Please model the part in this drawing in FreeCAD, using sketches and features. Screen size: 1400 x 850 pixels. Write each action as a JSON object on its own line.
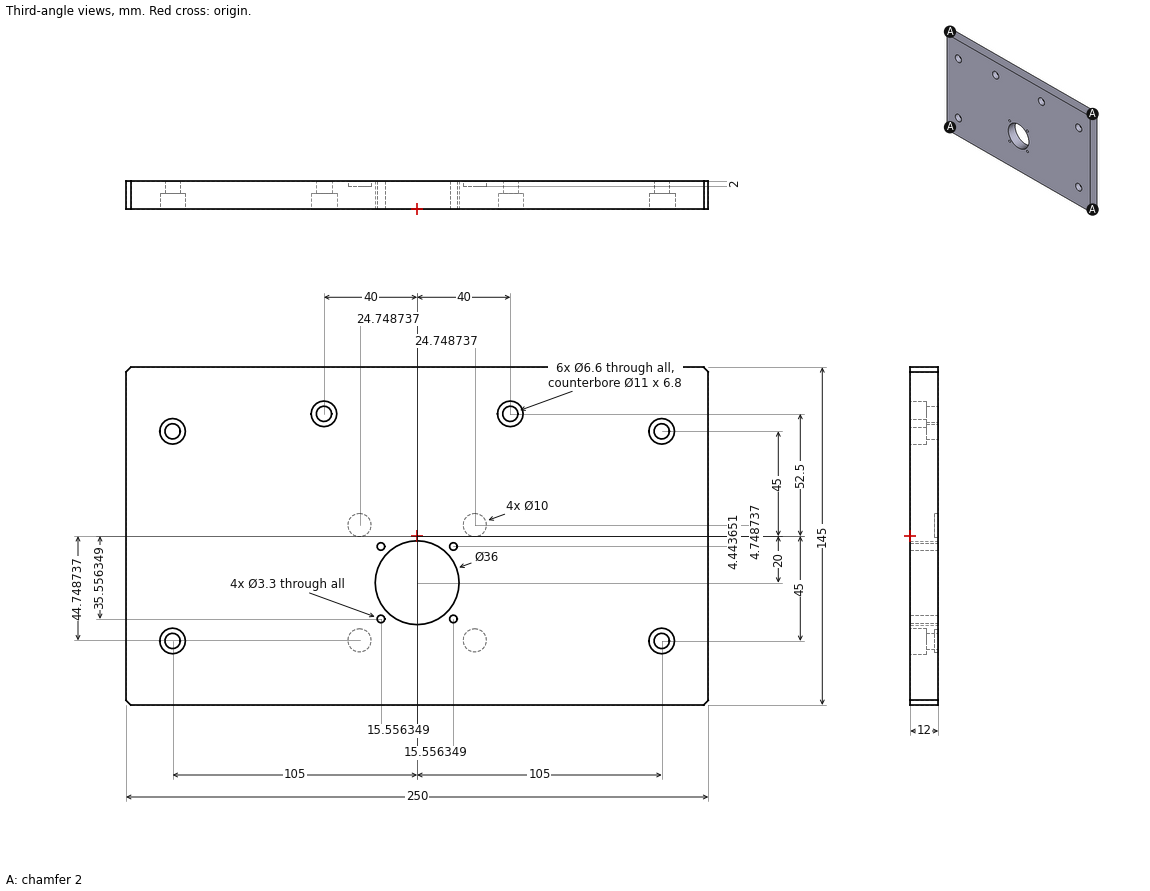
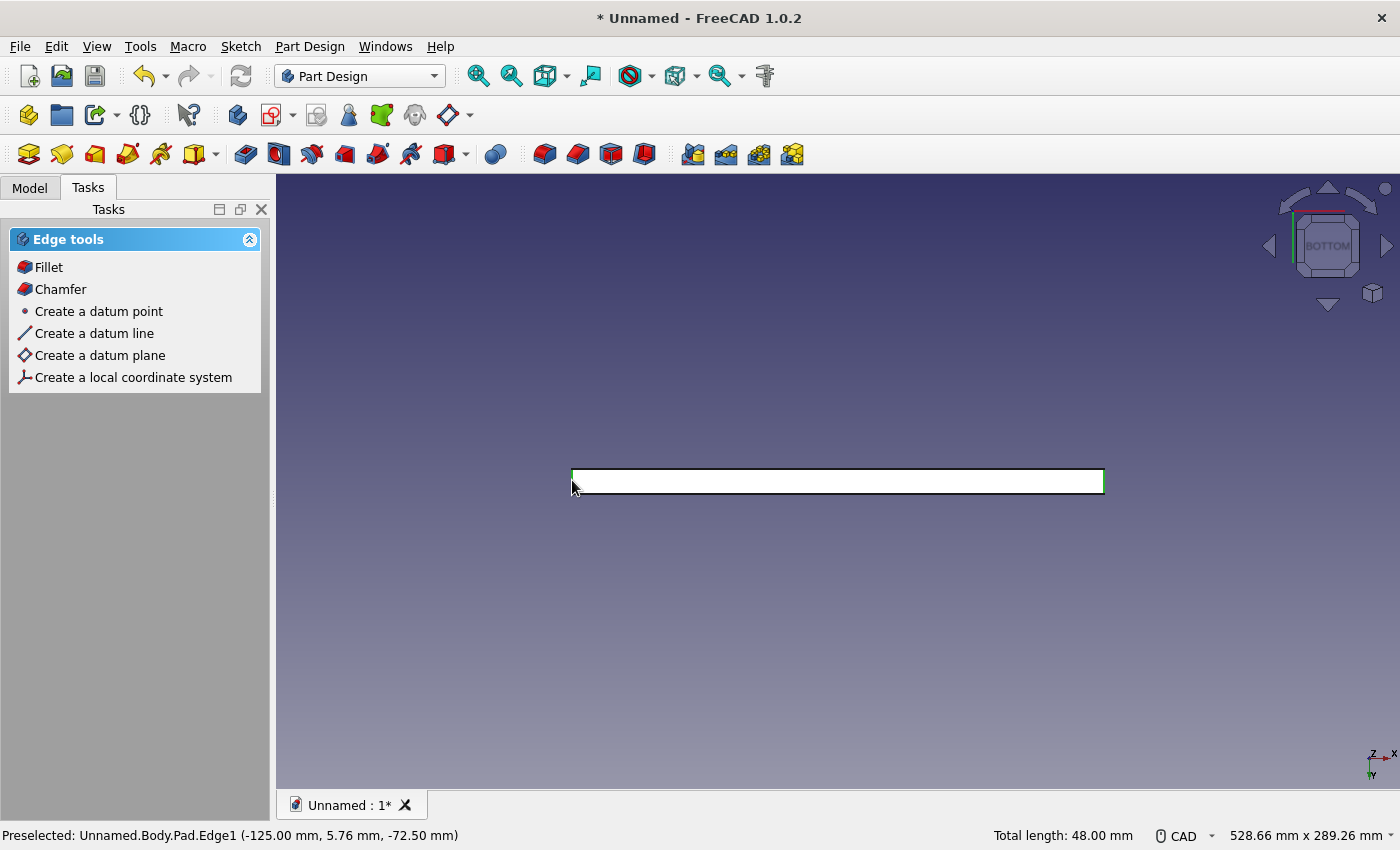
{"action": "left_click", "coordinate": [578, 154]}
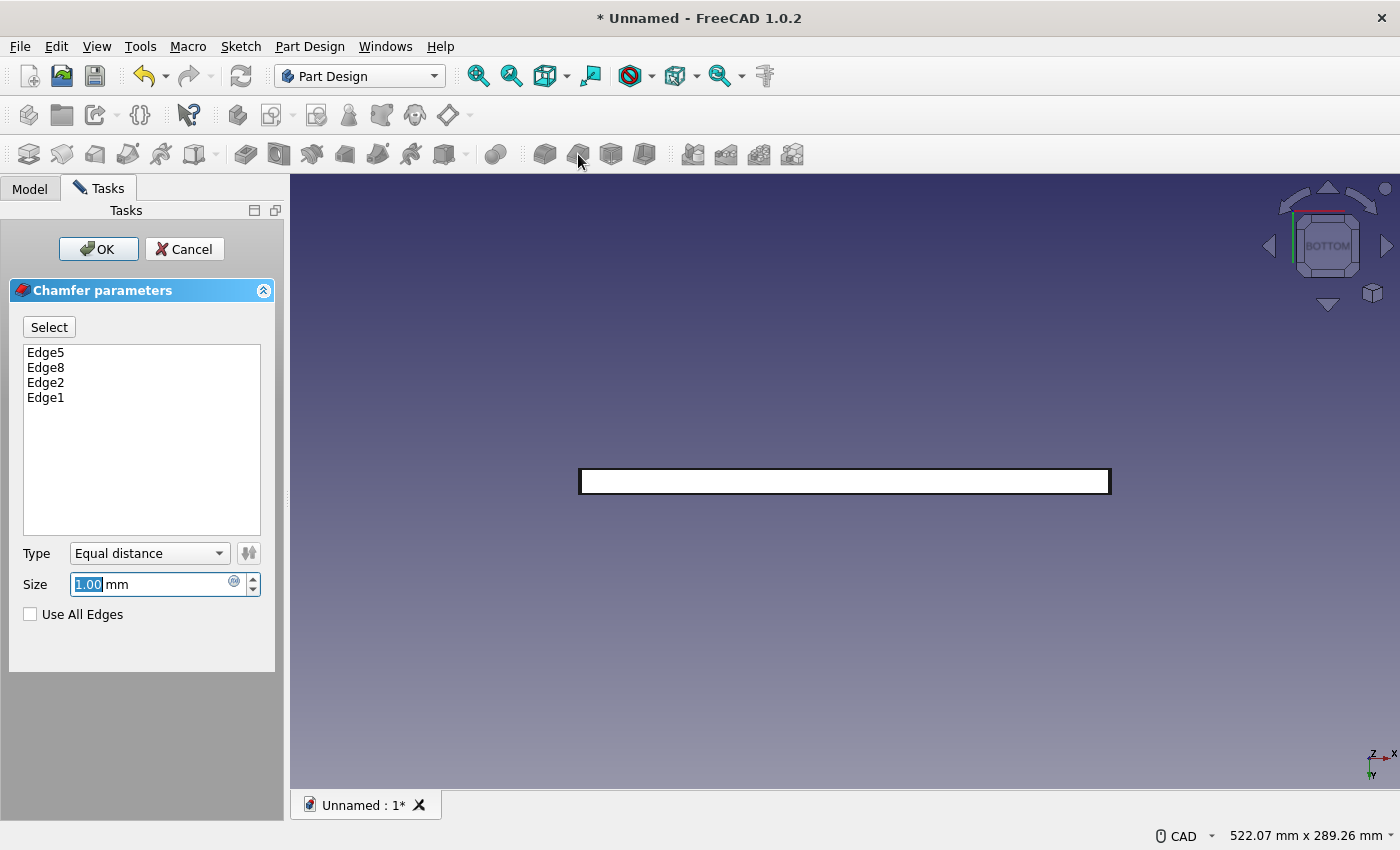
{"action": "type", "text": "2"}
{"action": "key", "text": "Tab"}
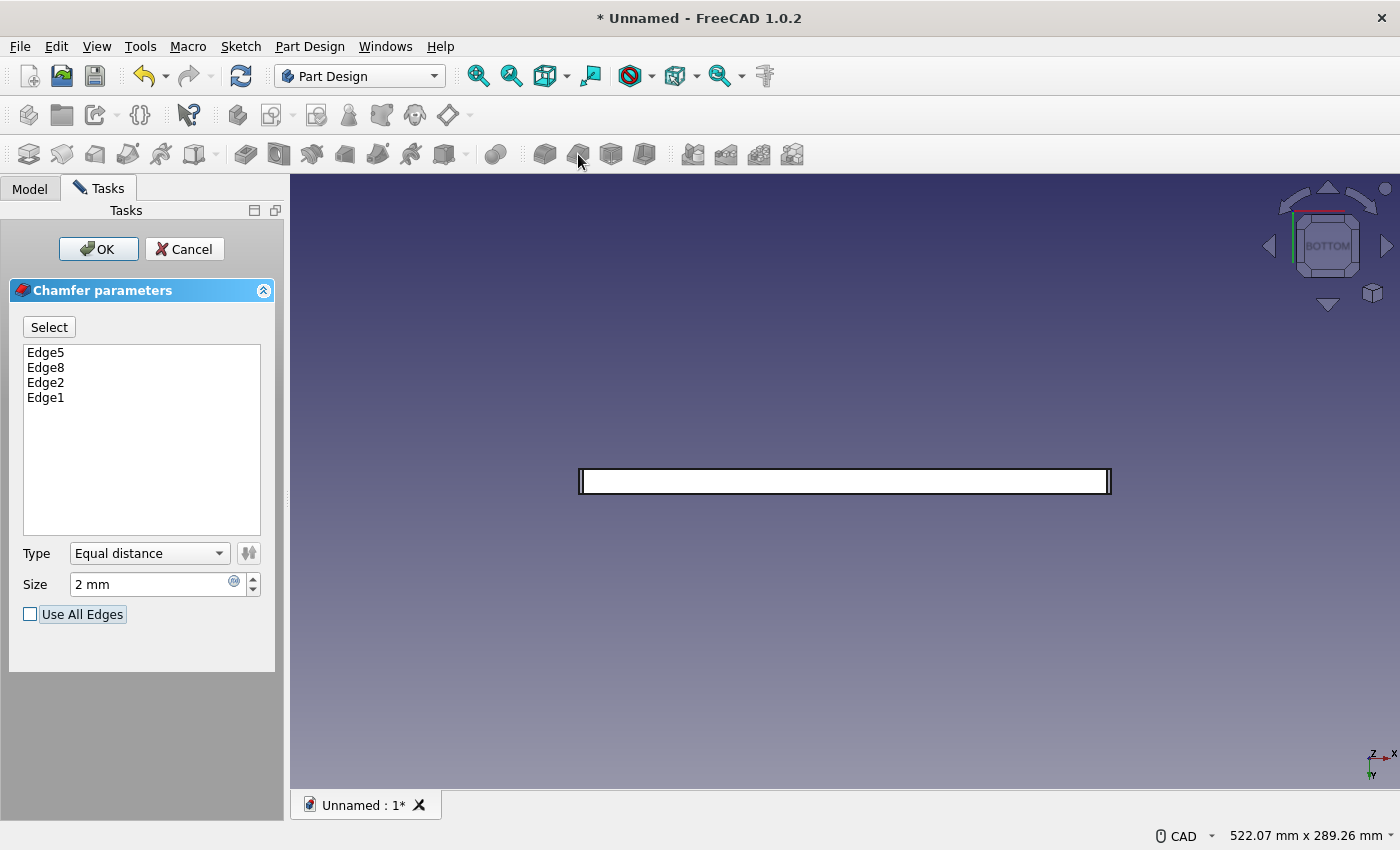
{"action": "left_click", "coordinate": [99, 249]}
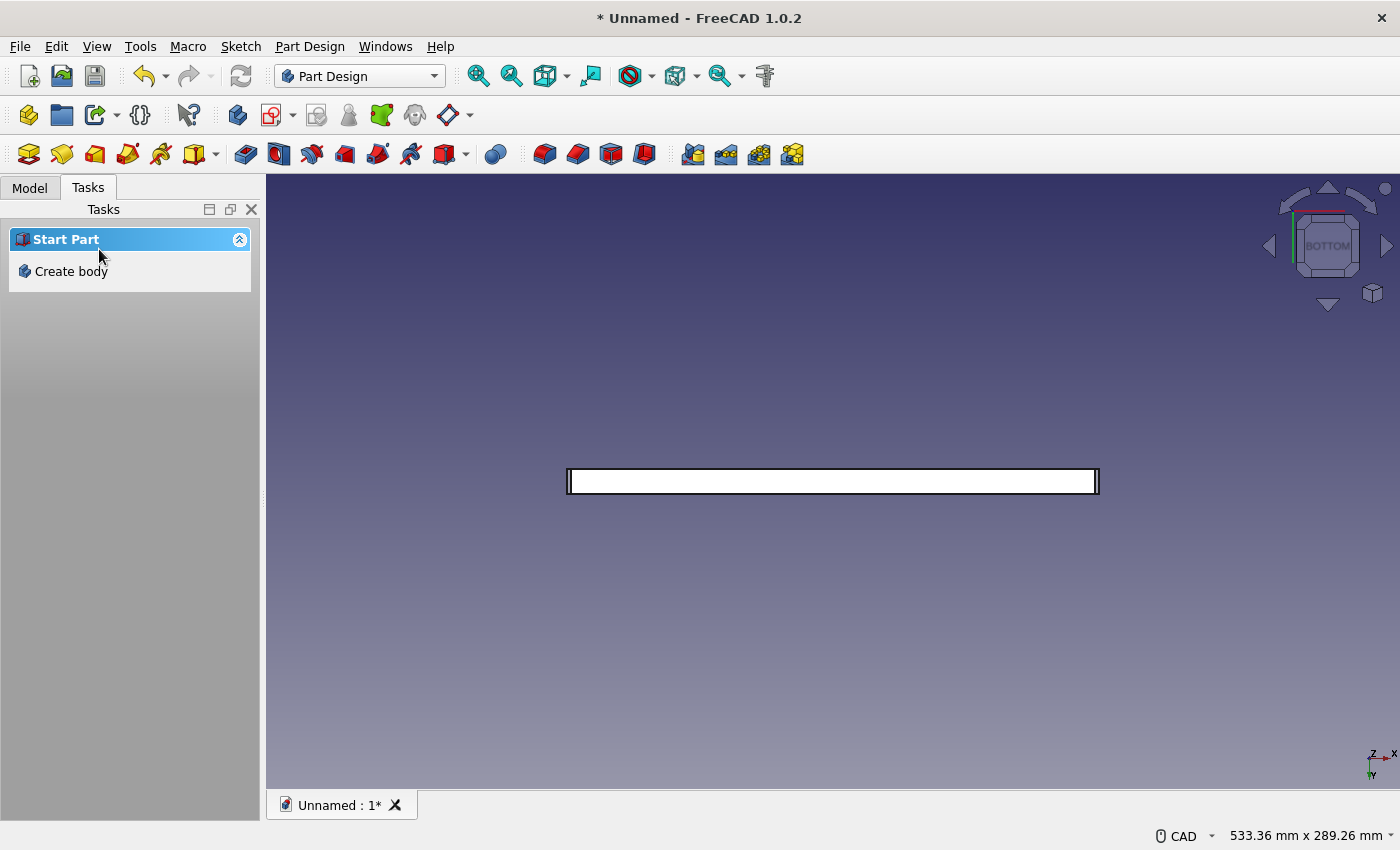
{"action": "key", "text": "4"}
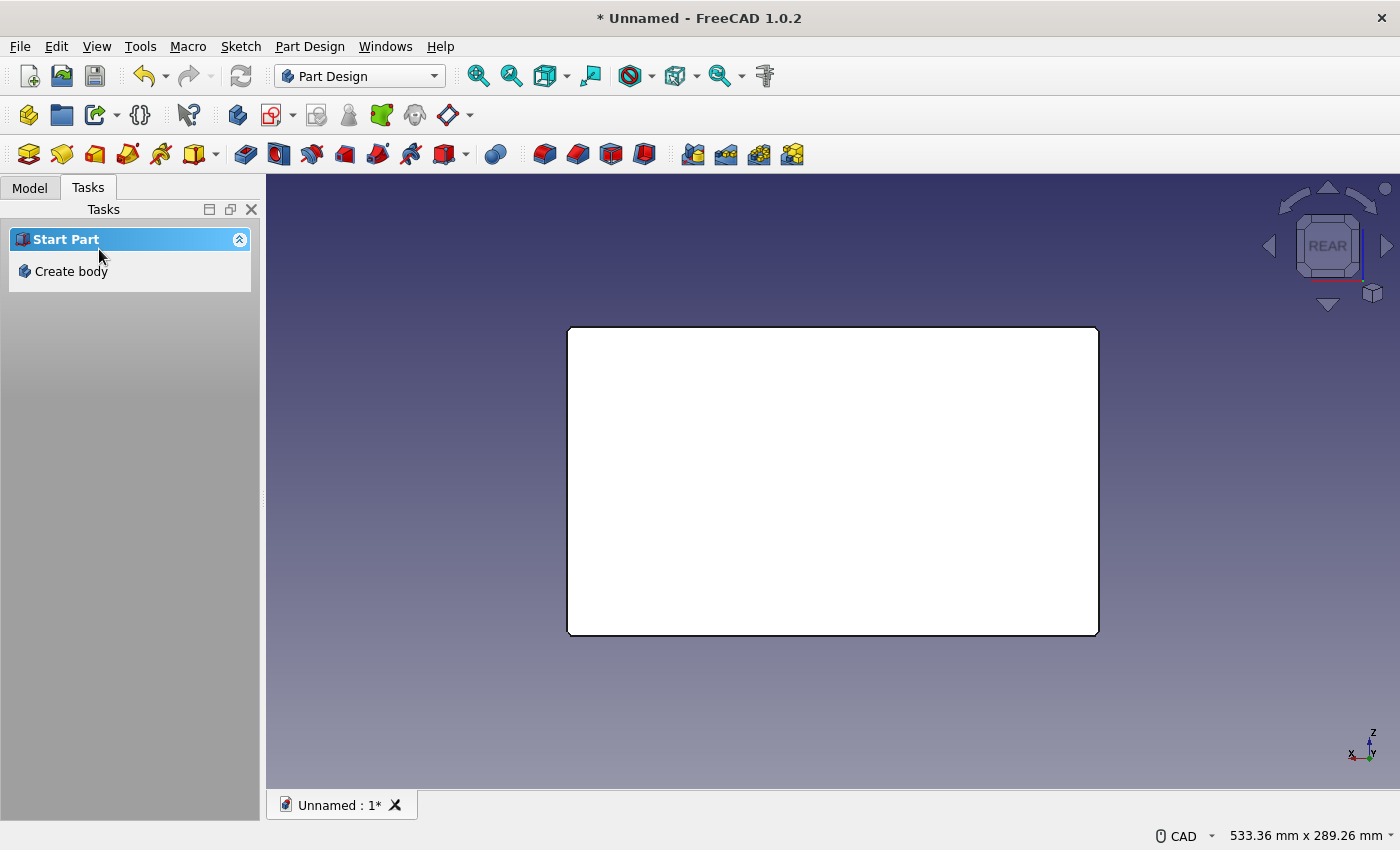
{"action": "left_click", "coordinate": [757, 480]}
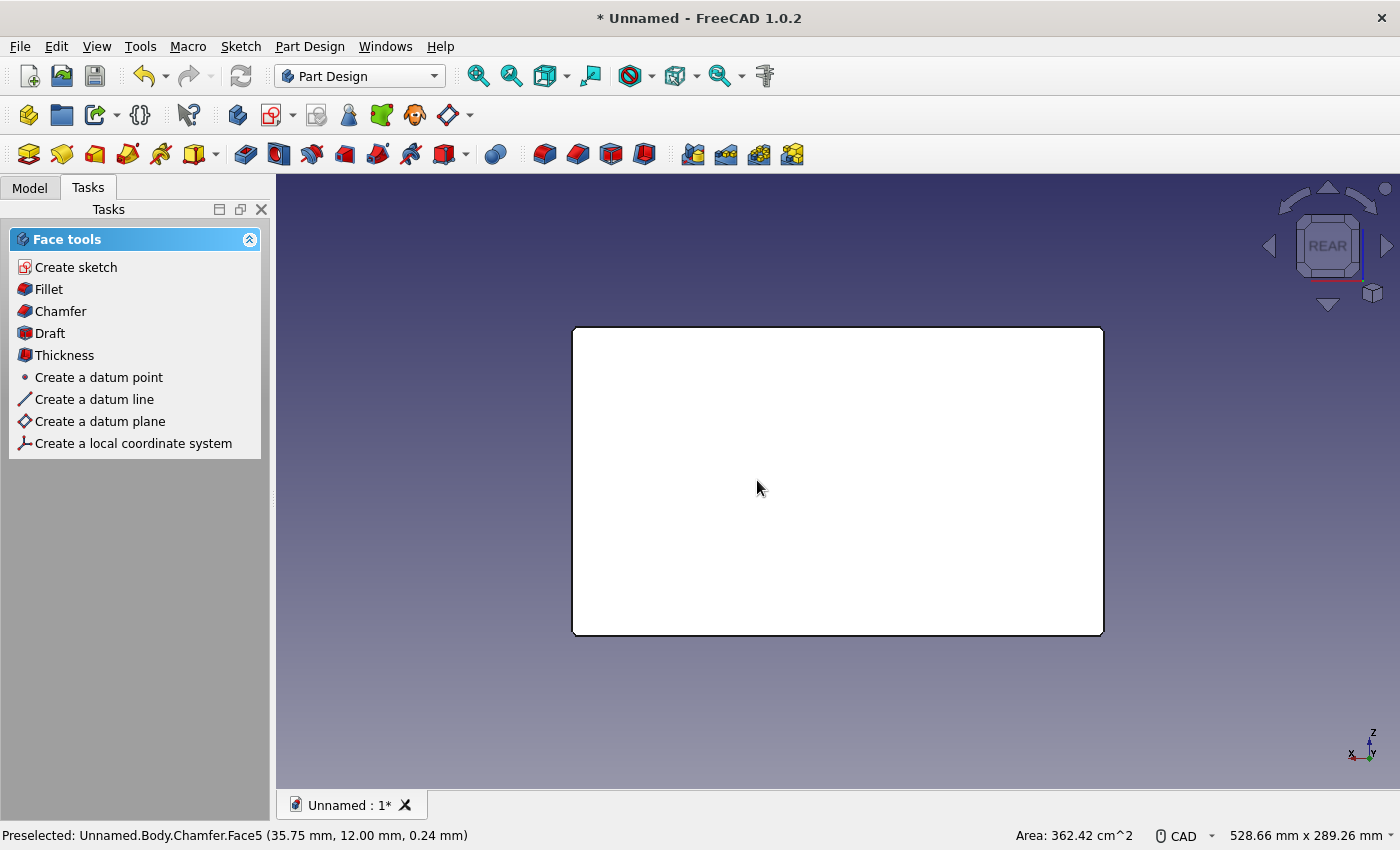
{"action": "left_click", "coordinate": [270, 116]}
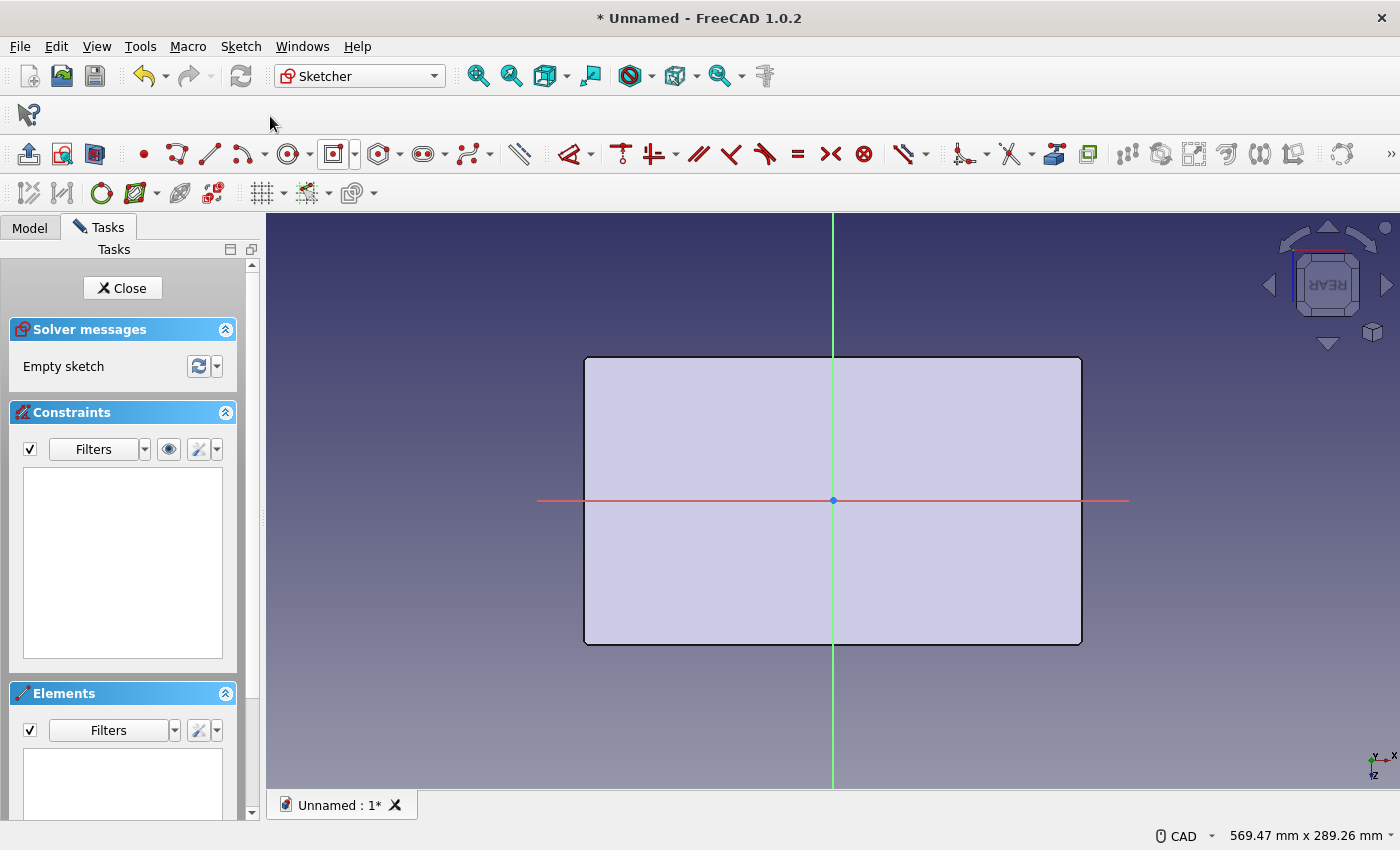
{"action": "scroll", "coordinate": [850, 454], "scroll_direction": "up", "scroll_amount": 8}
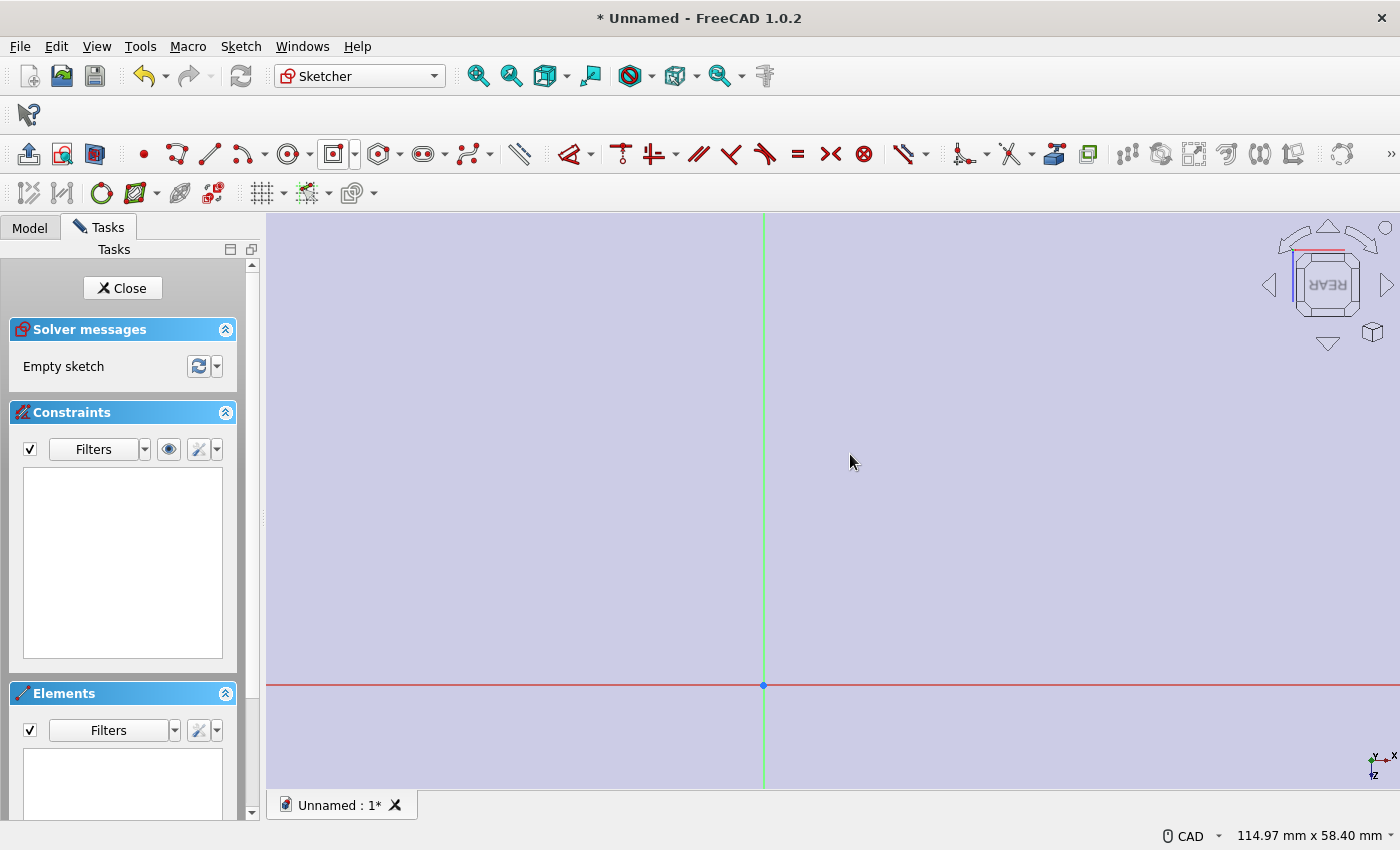
{"action": "left_click", "coordinate": [288, 154]}